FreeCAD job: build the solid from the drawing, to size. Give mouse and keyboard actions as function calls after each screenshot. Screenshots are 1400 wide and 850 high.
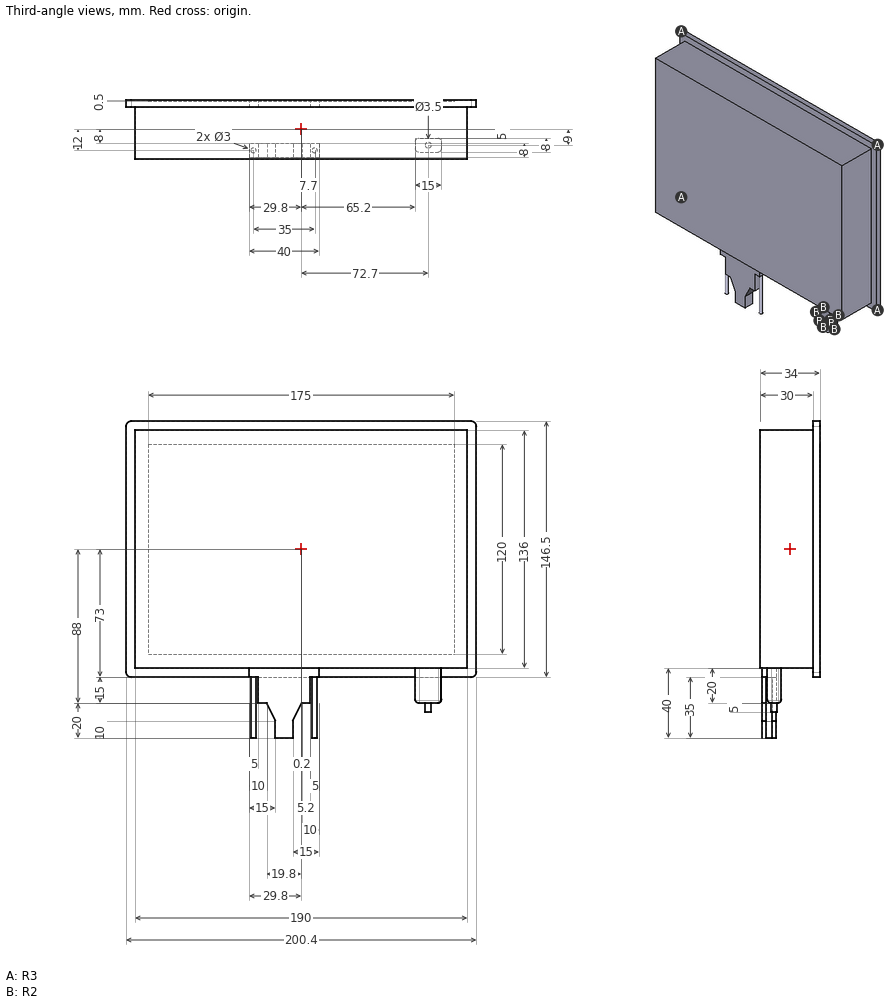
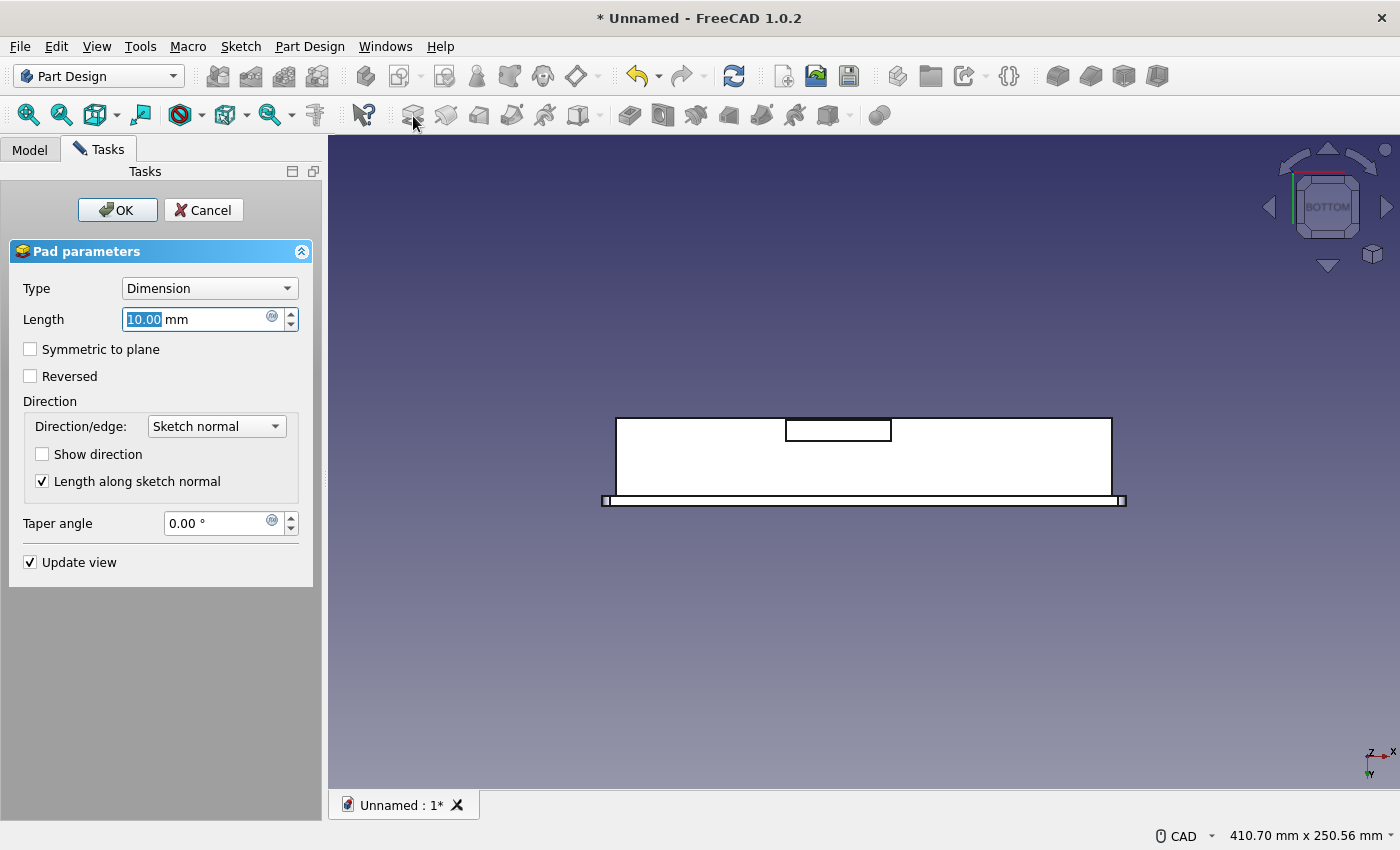
text(40)
key(Tab)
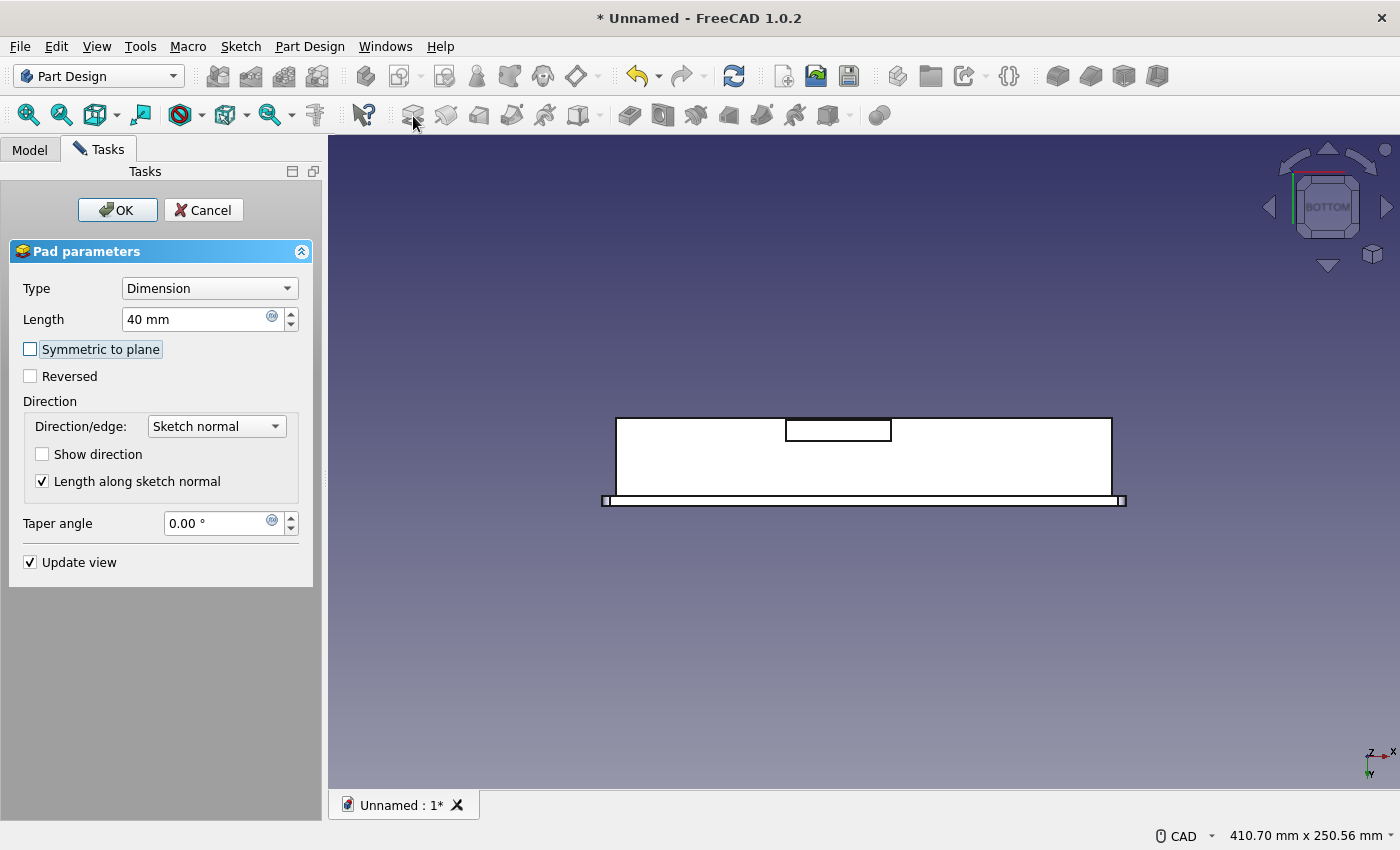
click(118, 210)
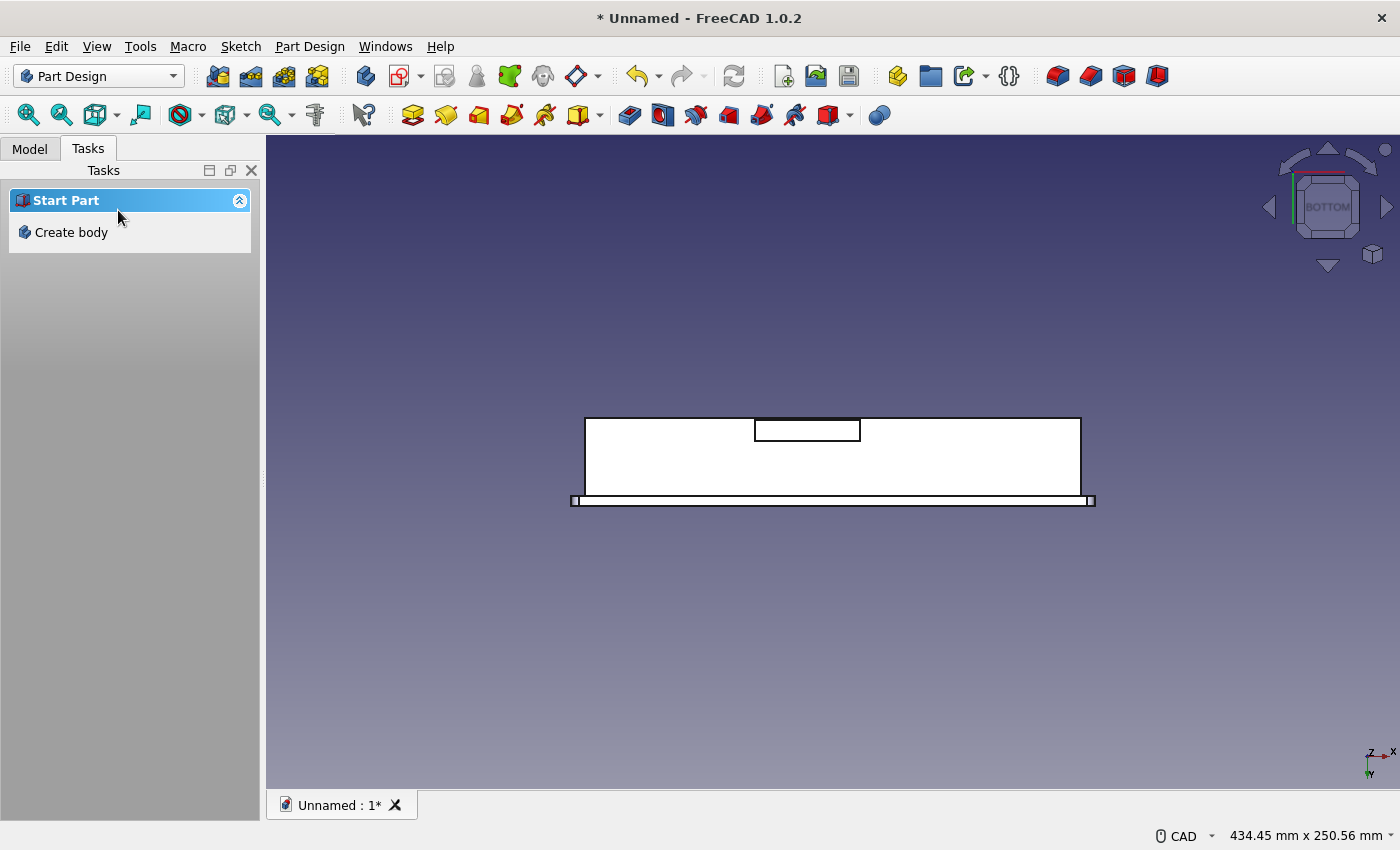
click(975, 456)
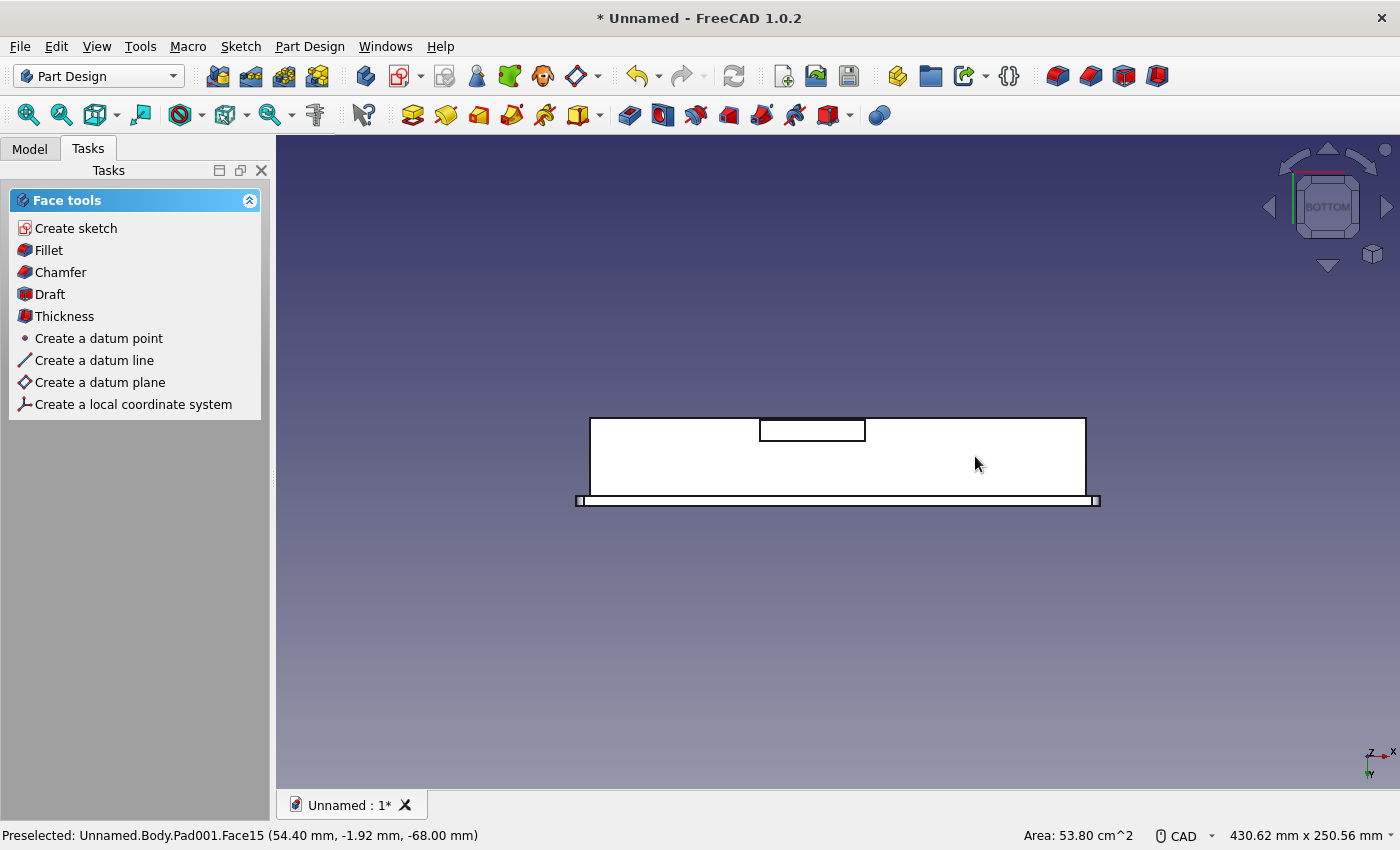
click(398, 76)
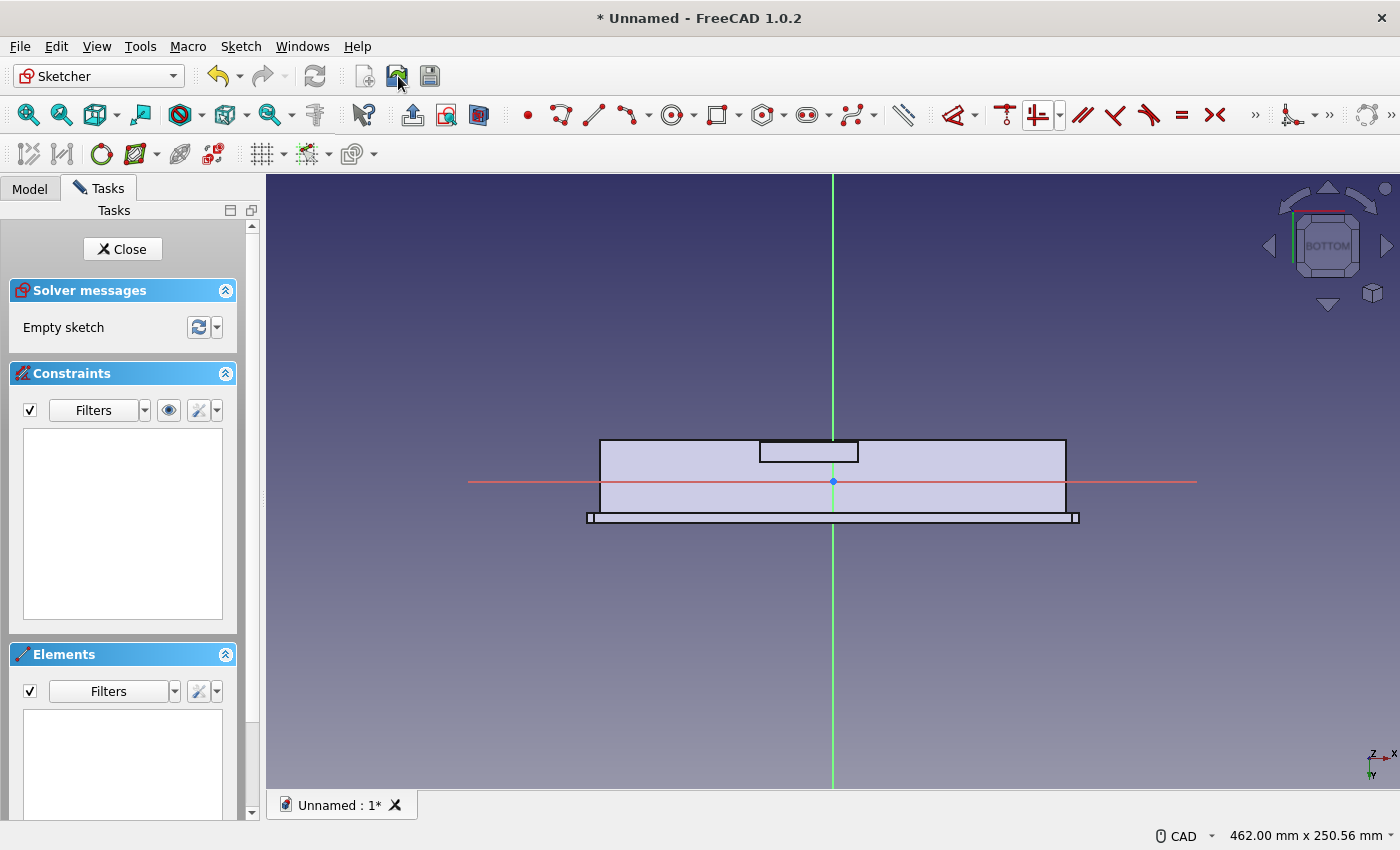
scroll(1027, 458, up, 14)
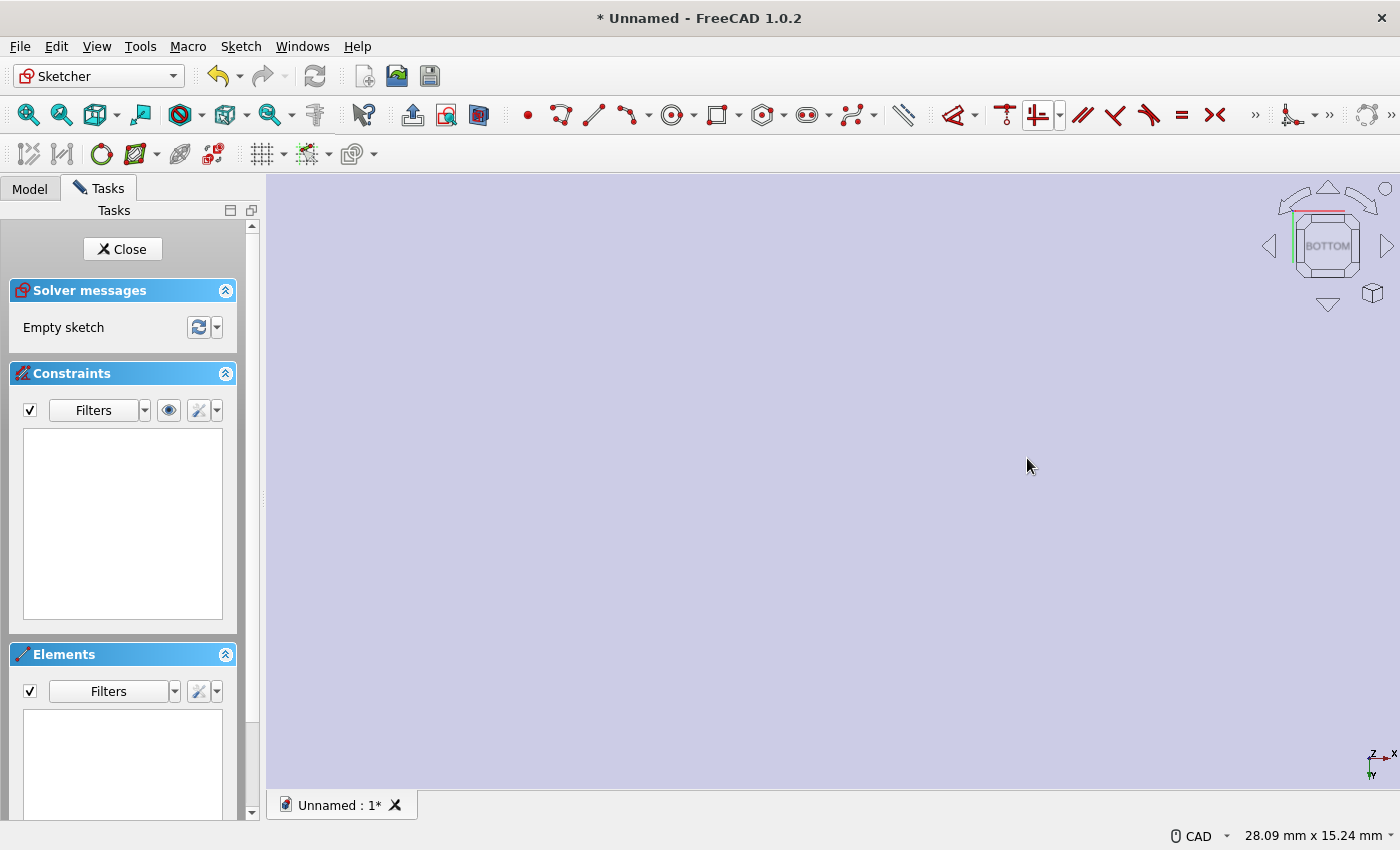
click(716, 116)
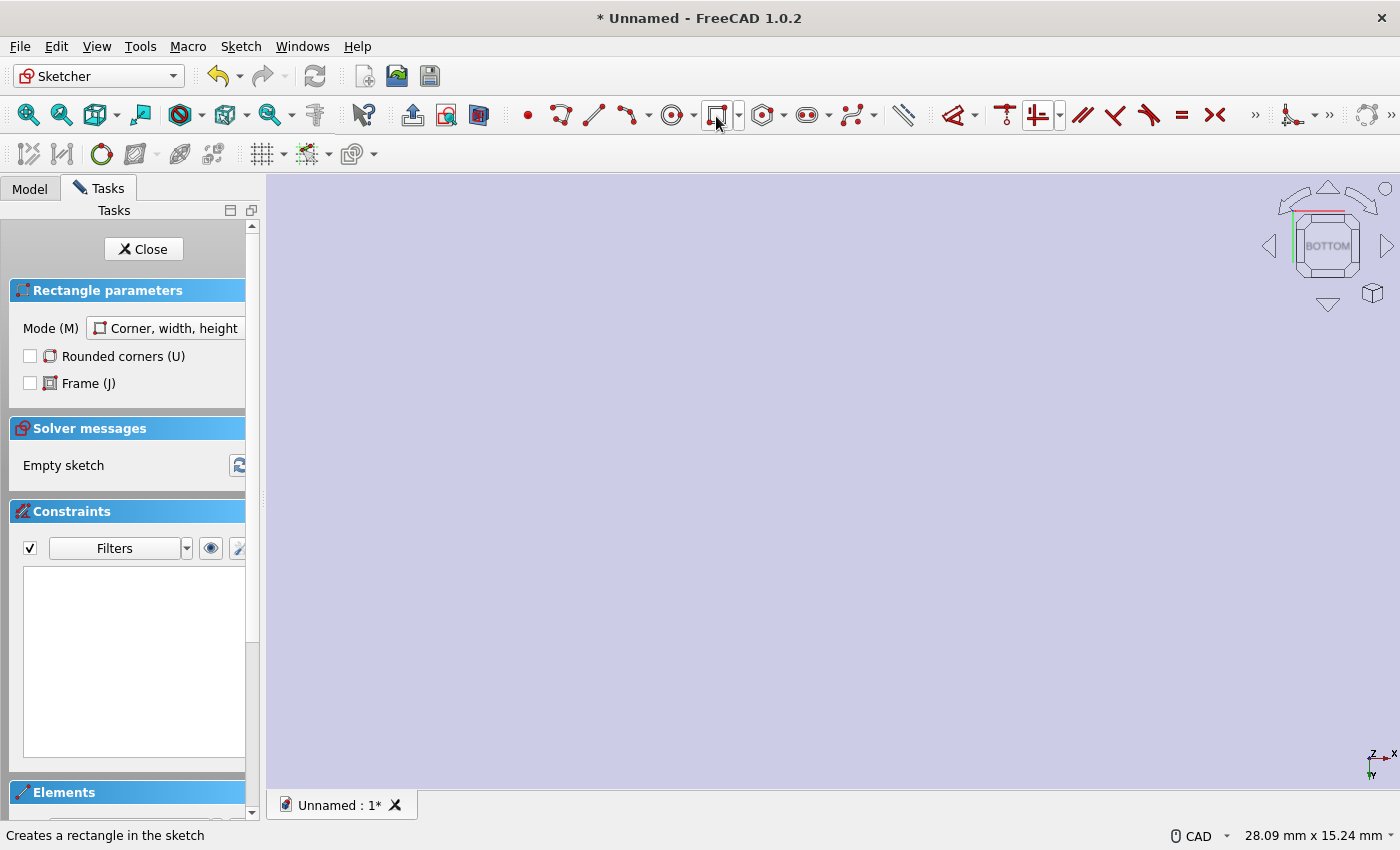
click(458, 313)
move(1064, 635)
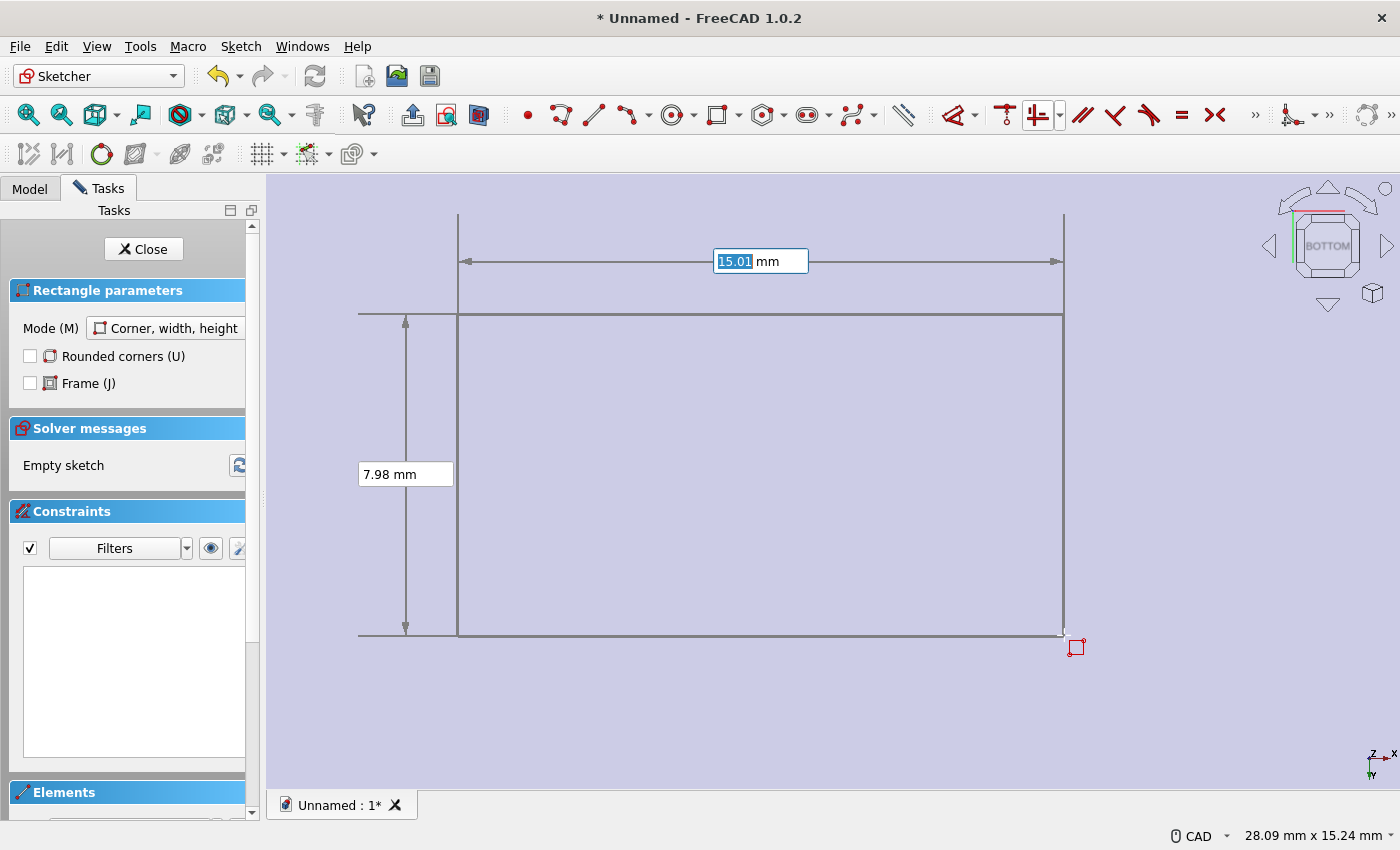
text(15)
key(Tab)
text(8)
key(Return)
key(Escape)